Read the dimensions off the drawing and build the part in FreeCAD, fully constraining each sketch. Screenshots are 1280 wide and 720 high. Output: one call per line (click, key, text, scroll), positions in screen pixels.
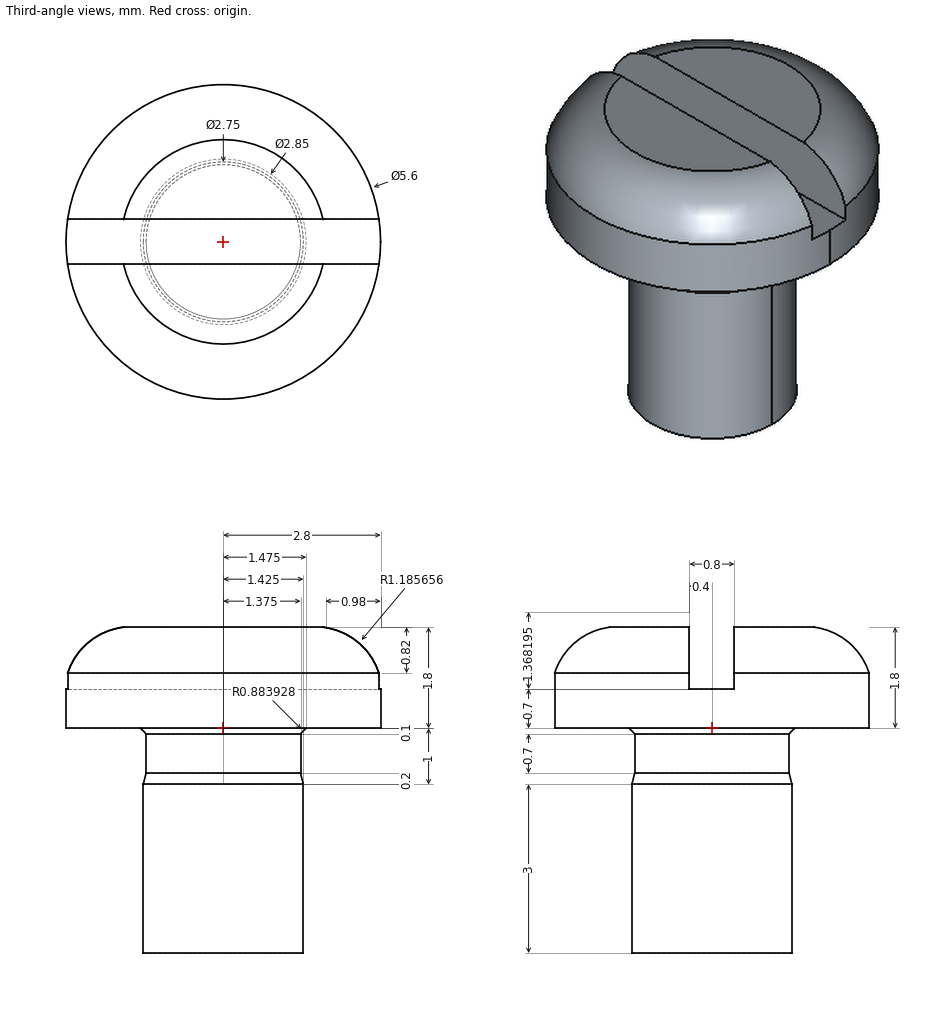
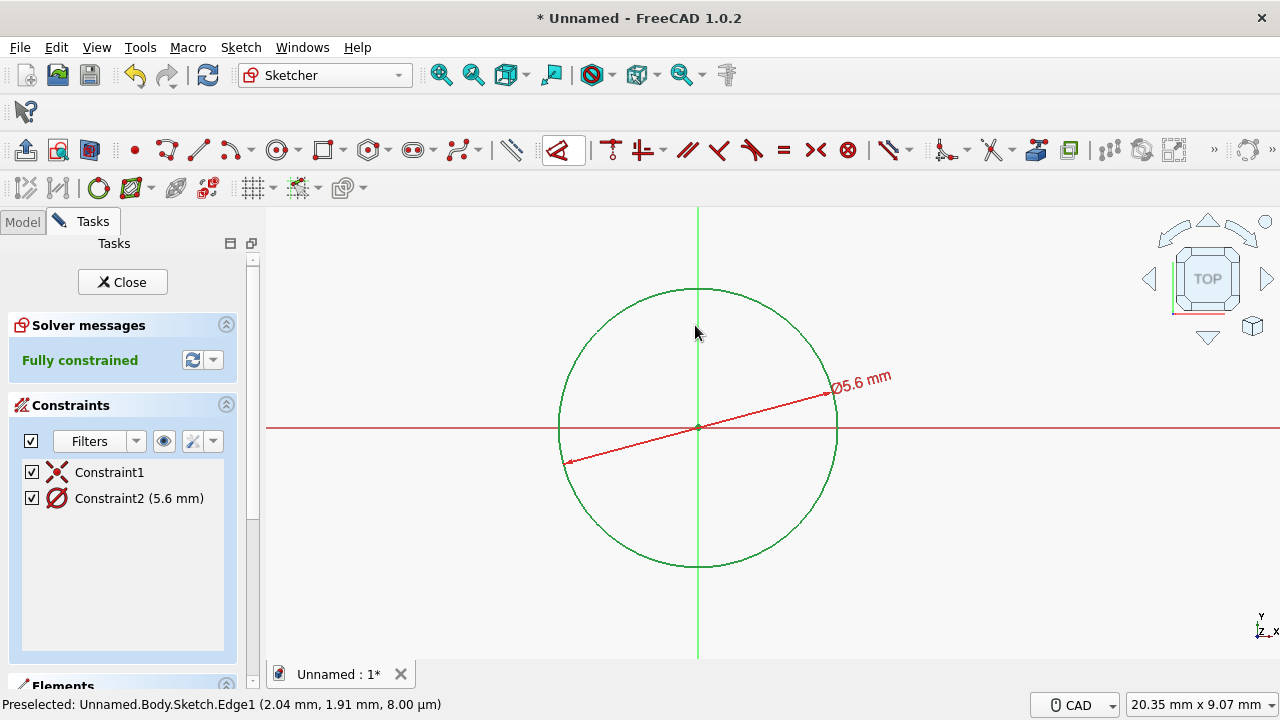
click(123, 282)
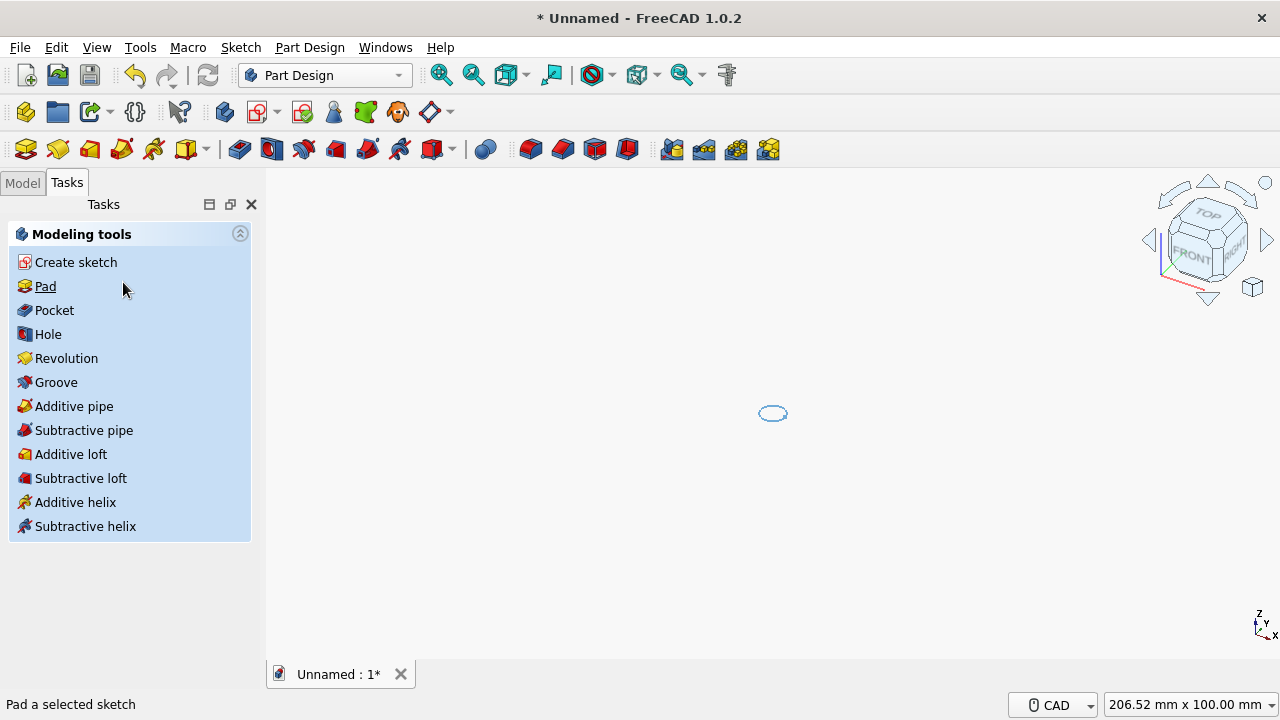
click(26, 150)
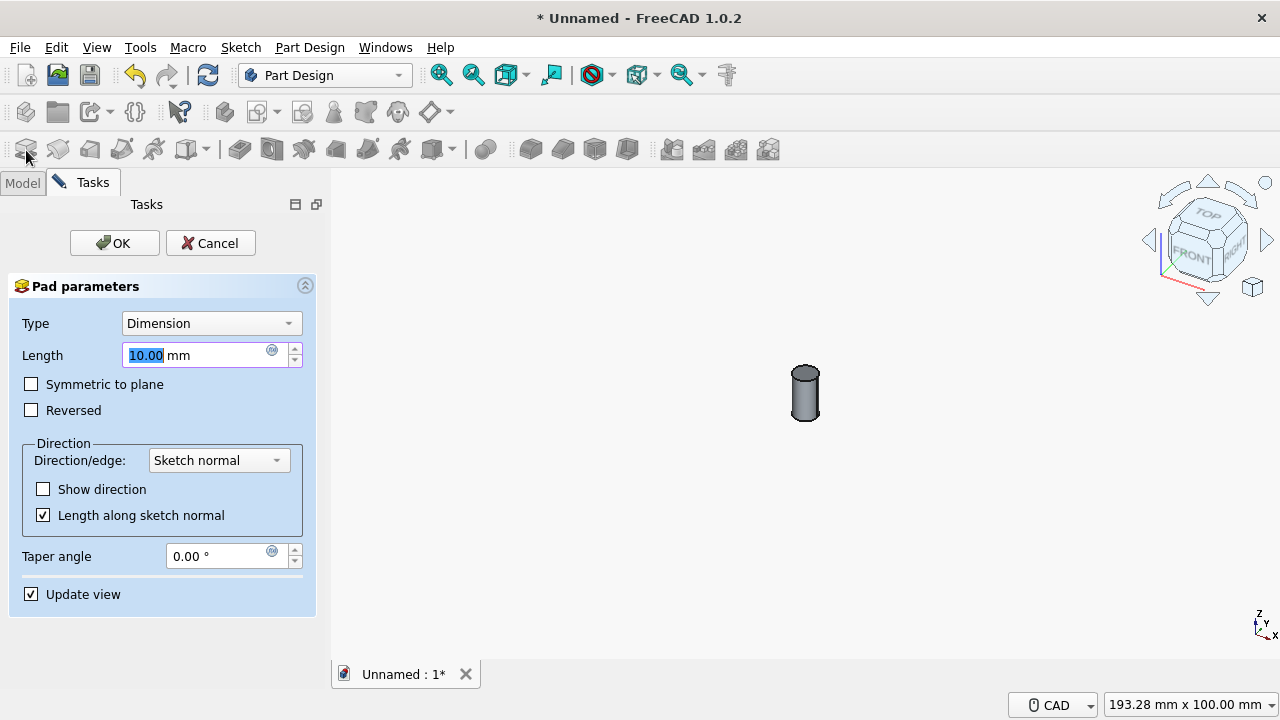
text(1.8)
key(Tab)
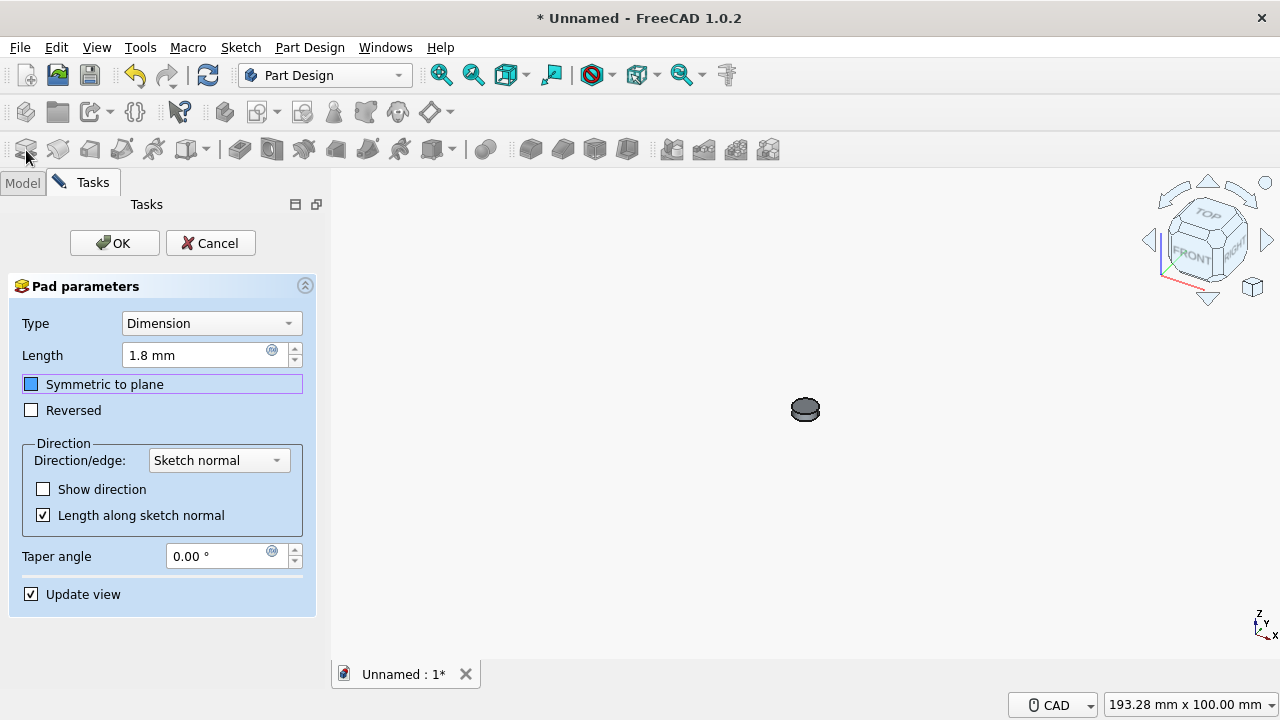
click(115, 243)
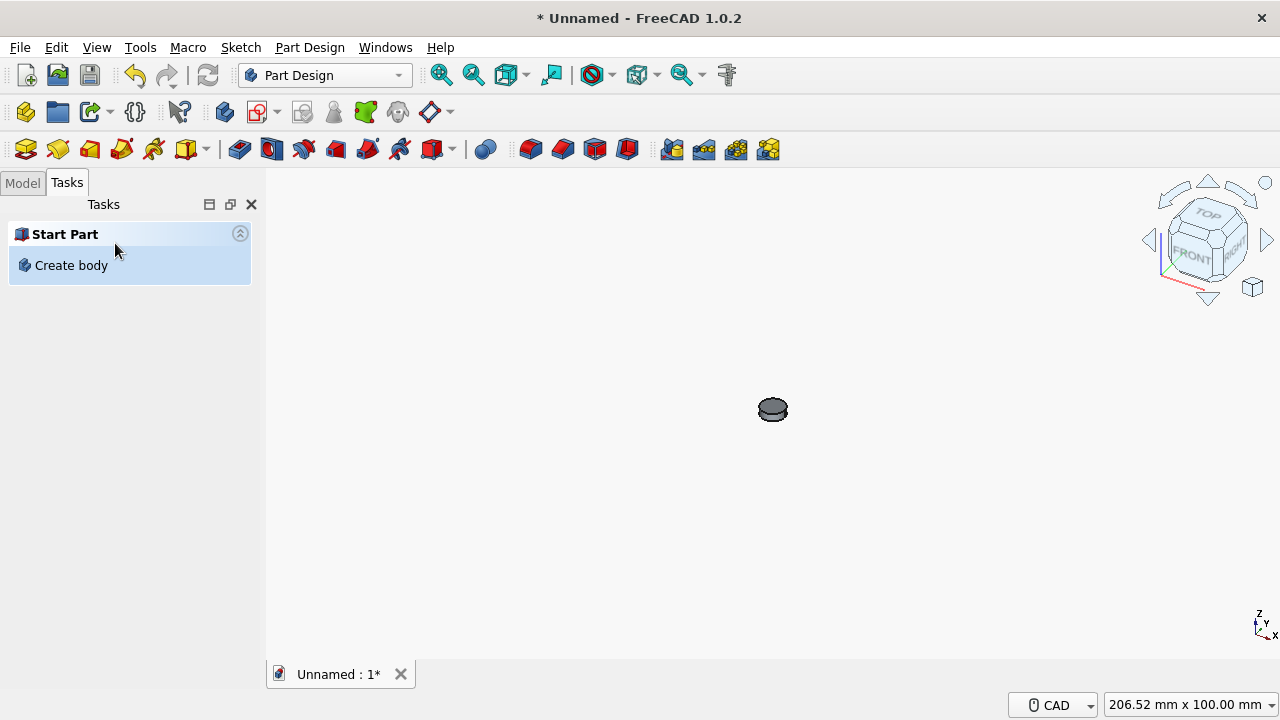
click(442, 76)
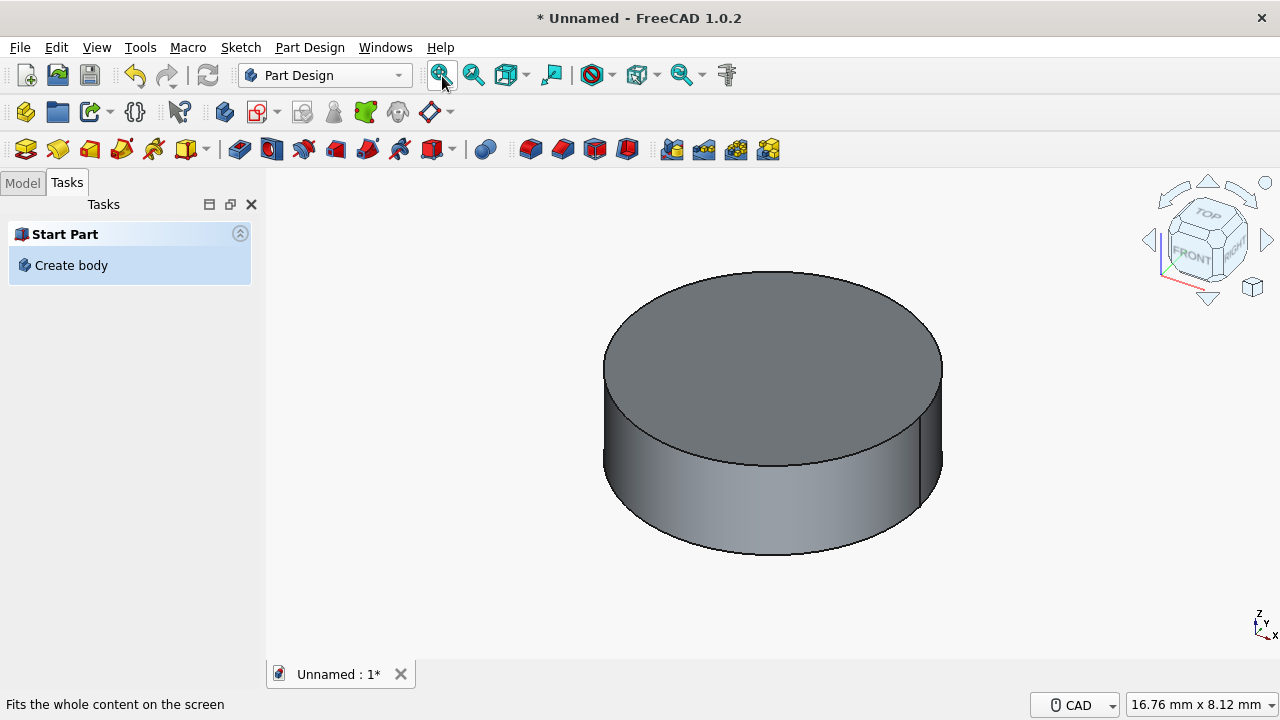
click(258, 112)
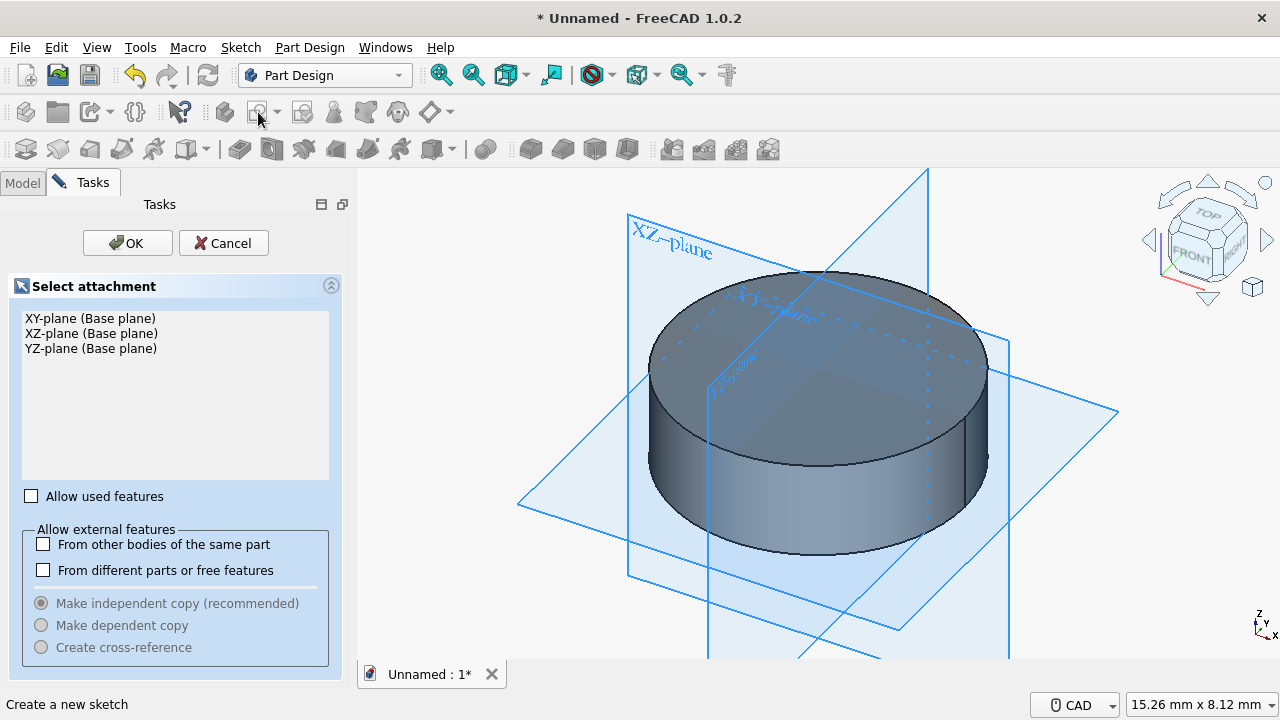
click(82, 334)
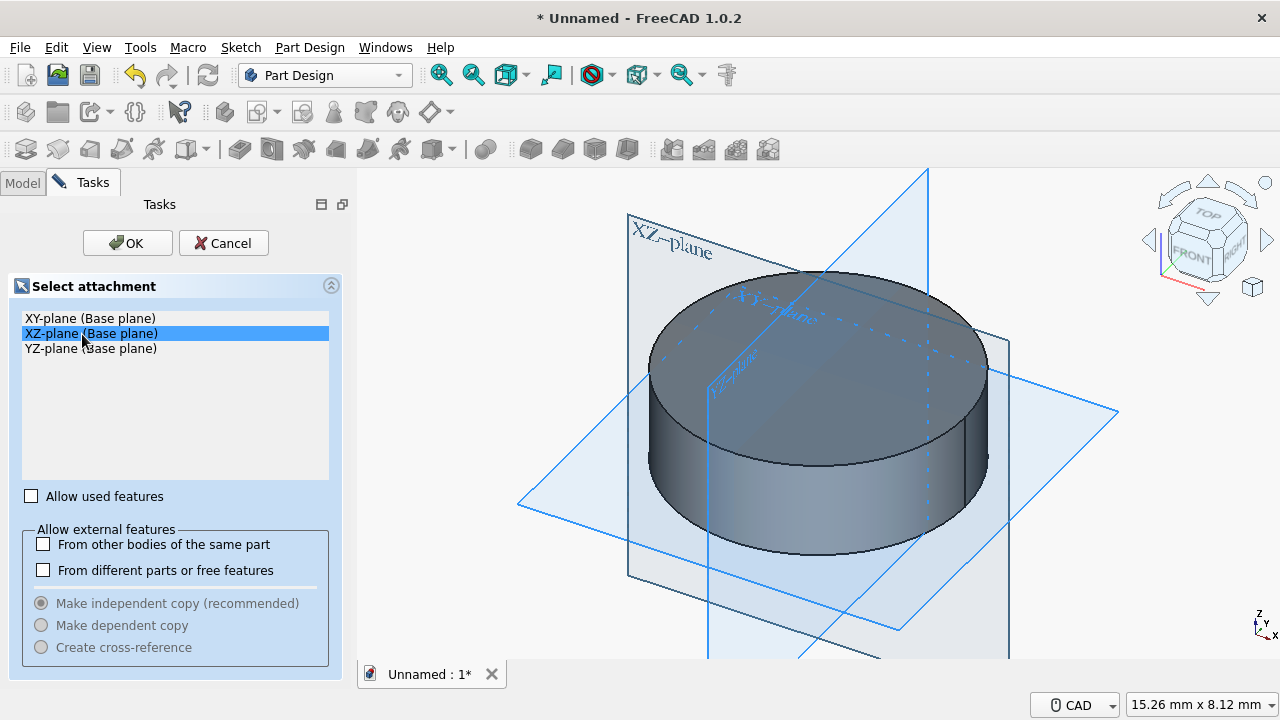
click(128, 243)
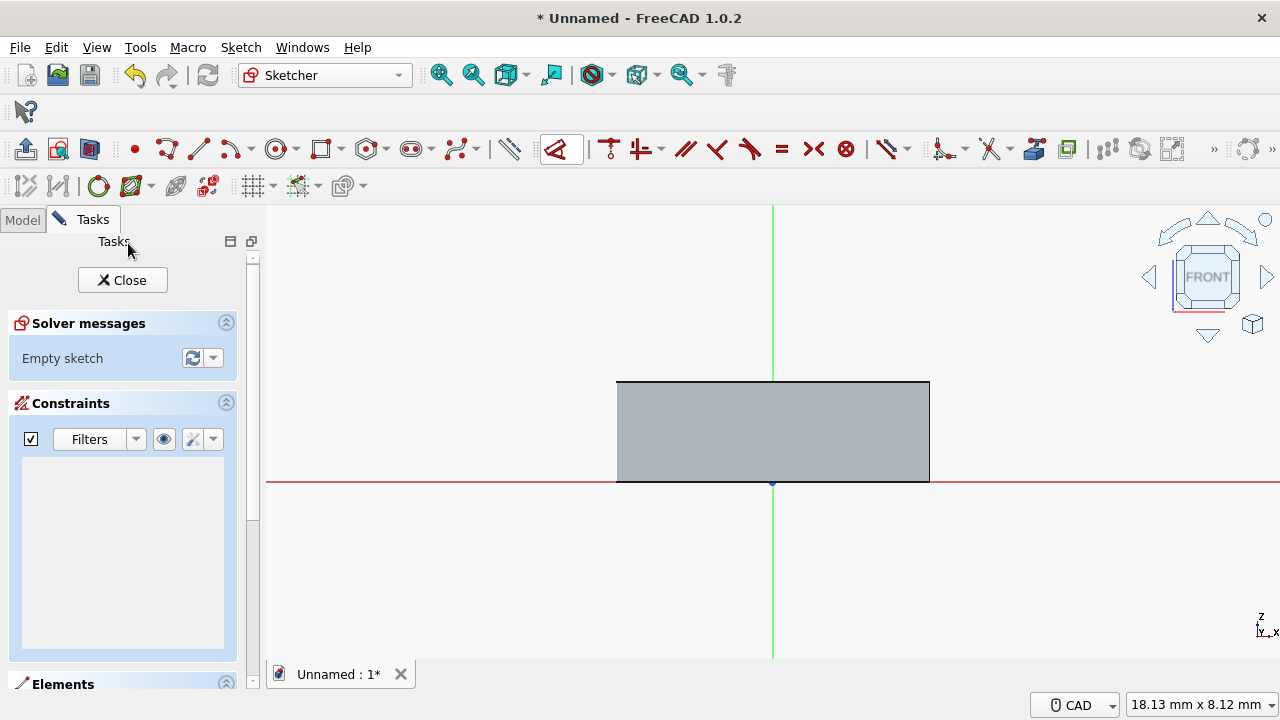
click(90, 150)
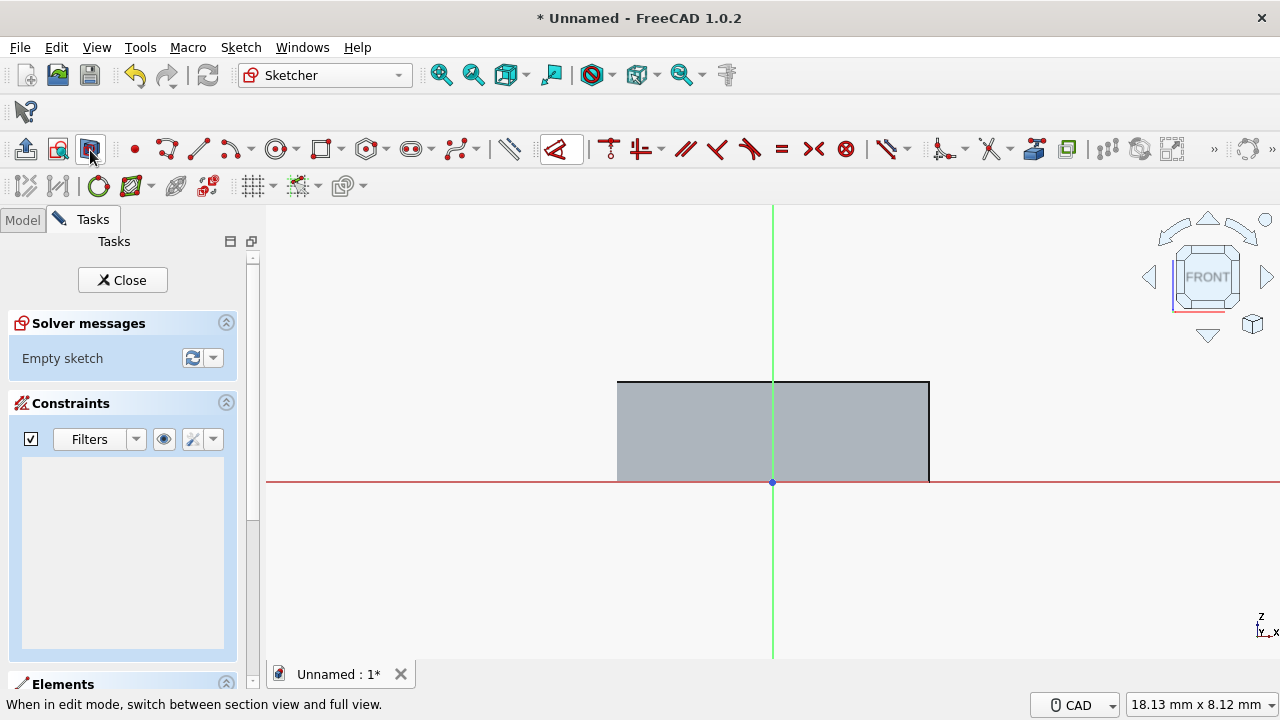
scroll(831, 493, up, 10)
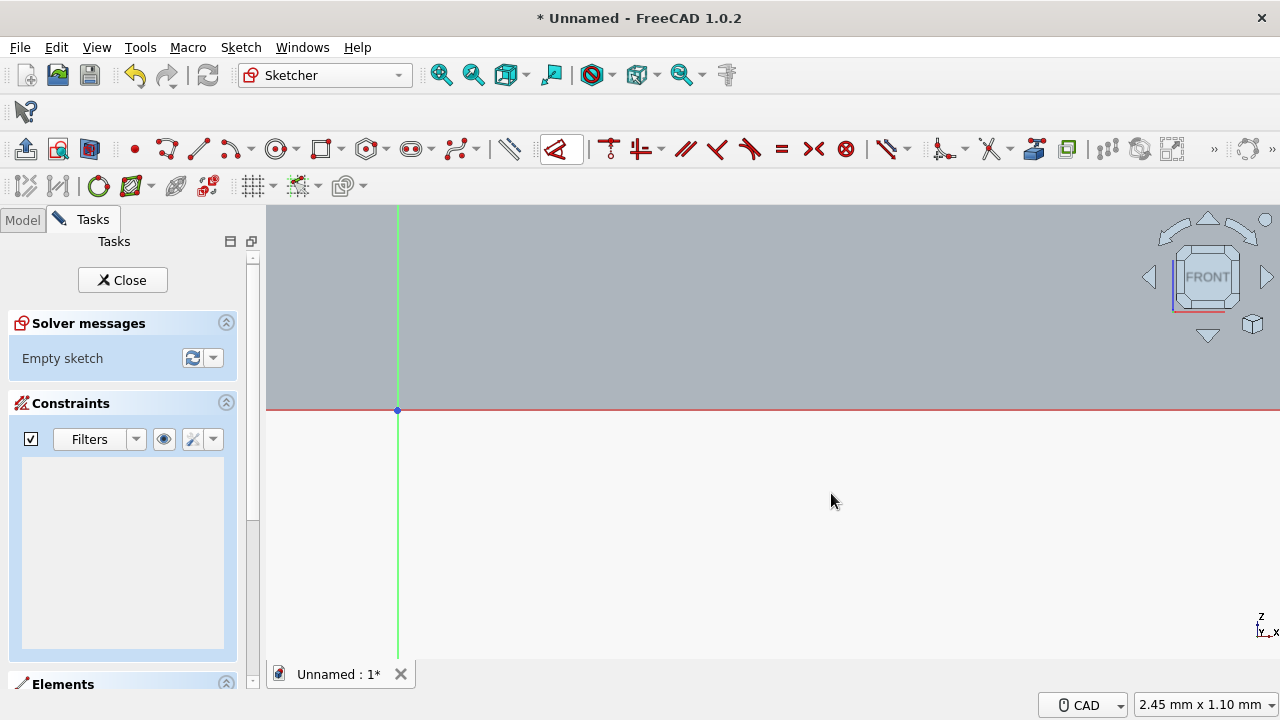
click(168, 150)